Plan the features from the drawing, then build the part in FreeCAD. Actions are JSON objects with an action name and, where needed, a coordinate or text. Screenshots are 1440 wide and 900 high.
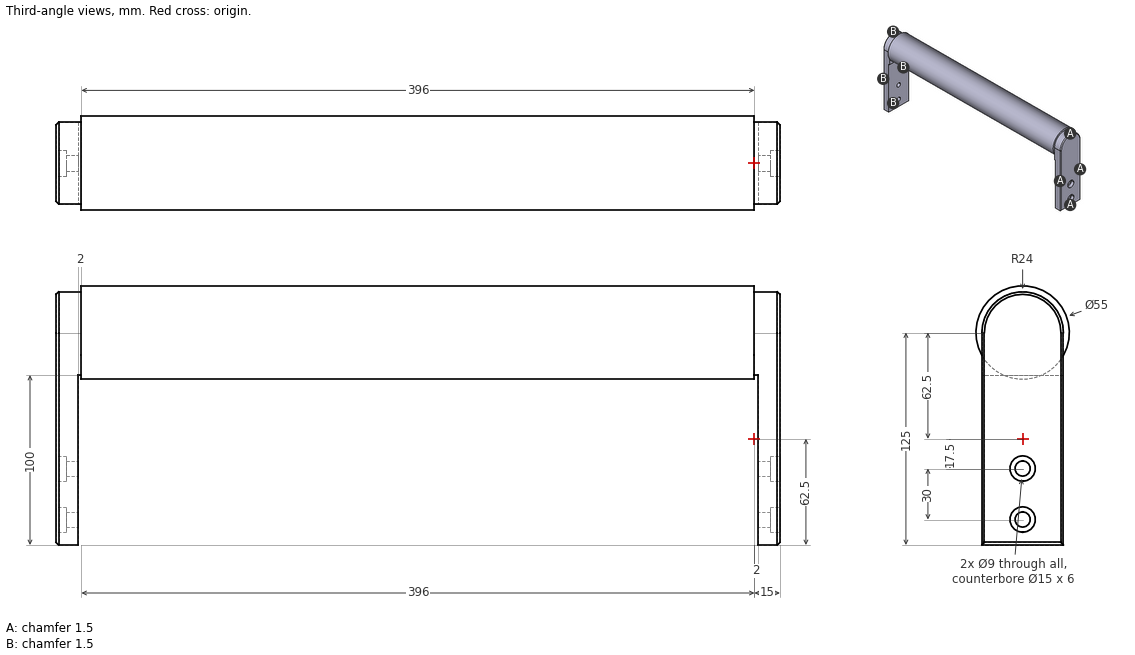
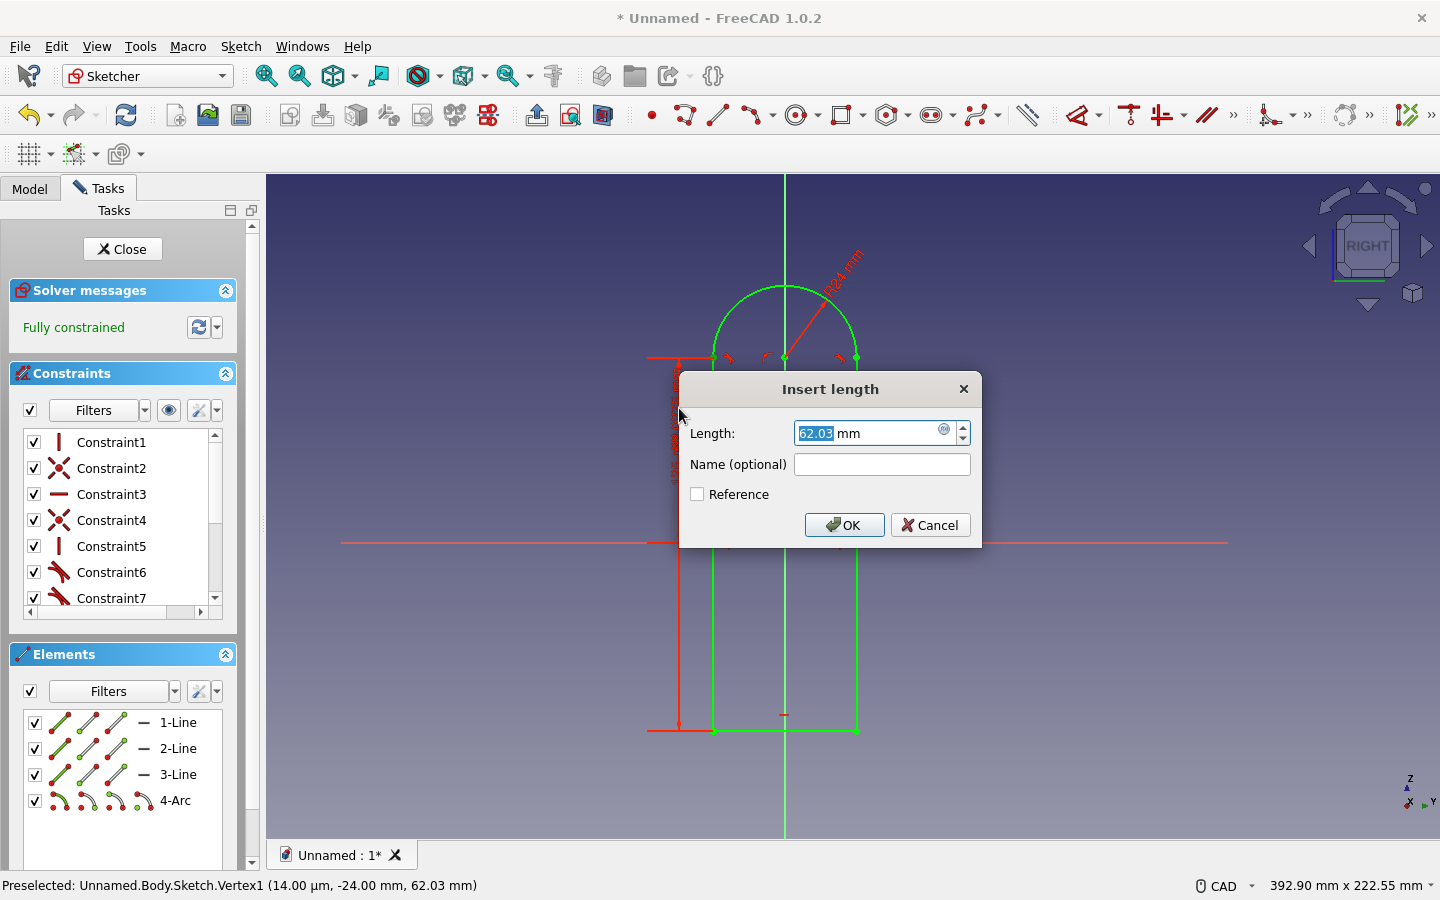
{"action": "type", "text": "62.5"}
{"action": "key", "text": "Return"}
{"action": "key", "text": "Escape"}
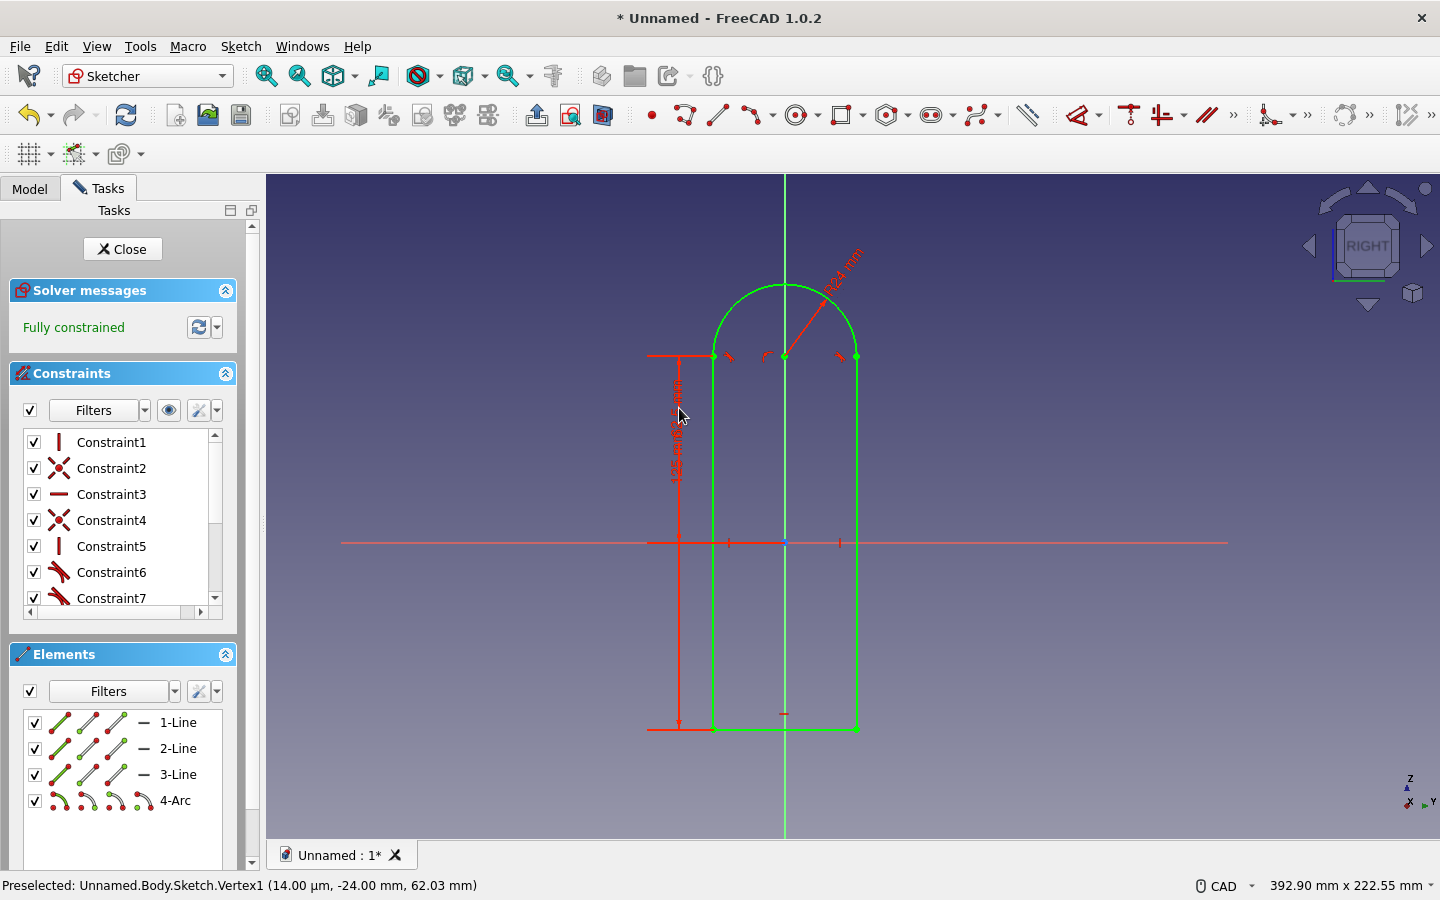
{"action": "left_click", "coordinate": [123, 249]}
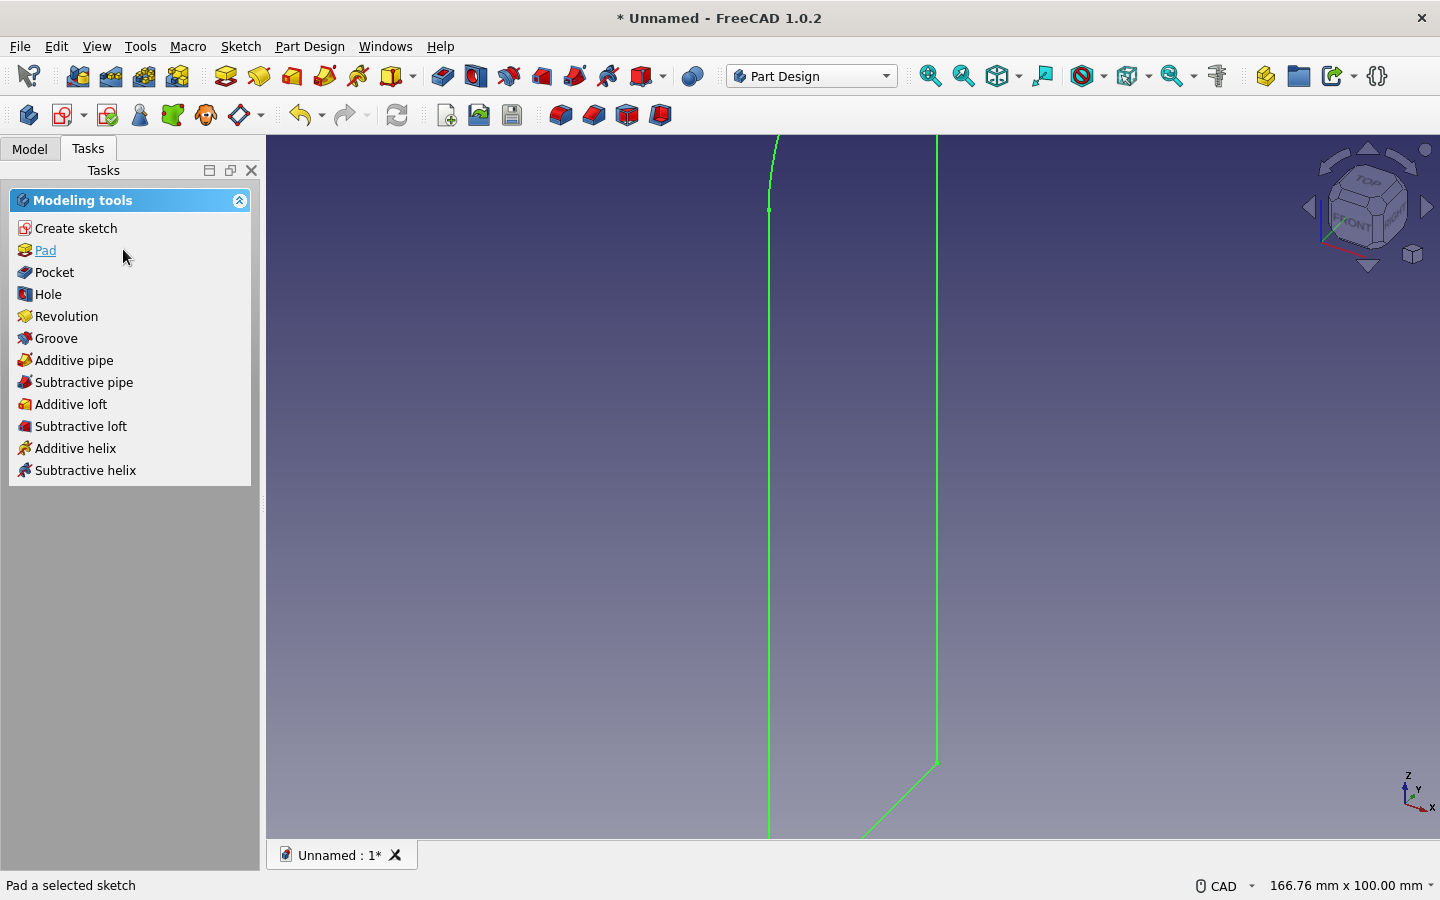
{"action": "left_click", "coordinate": [226, 76]}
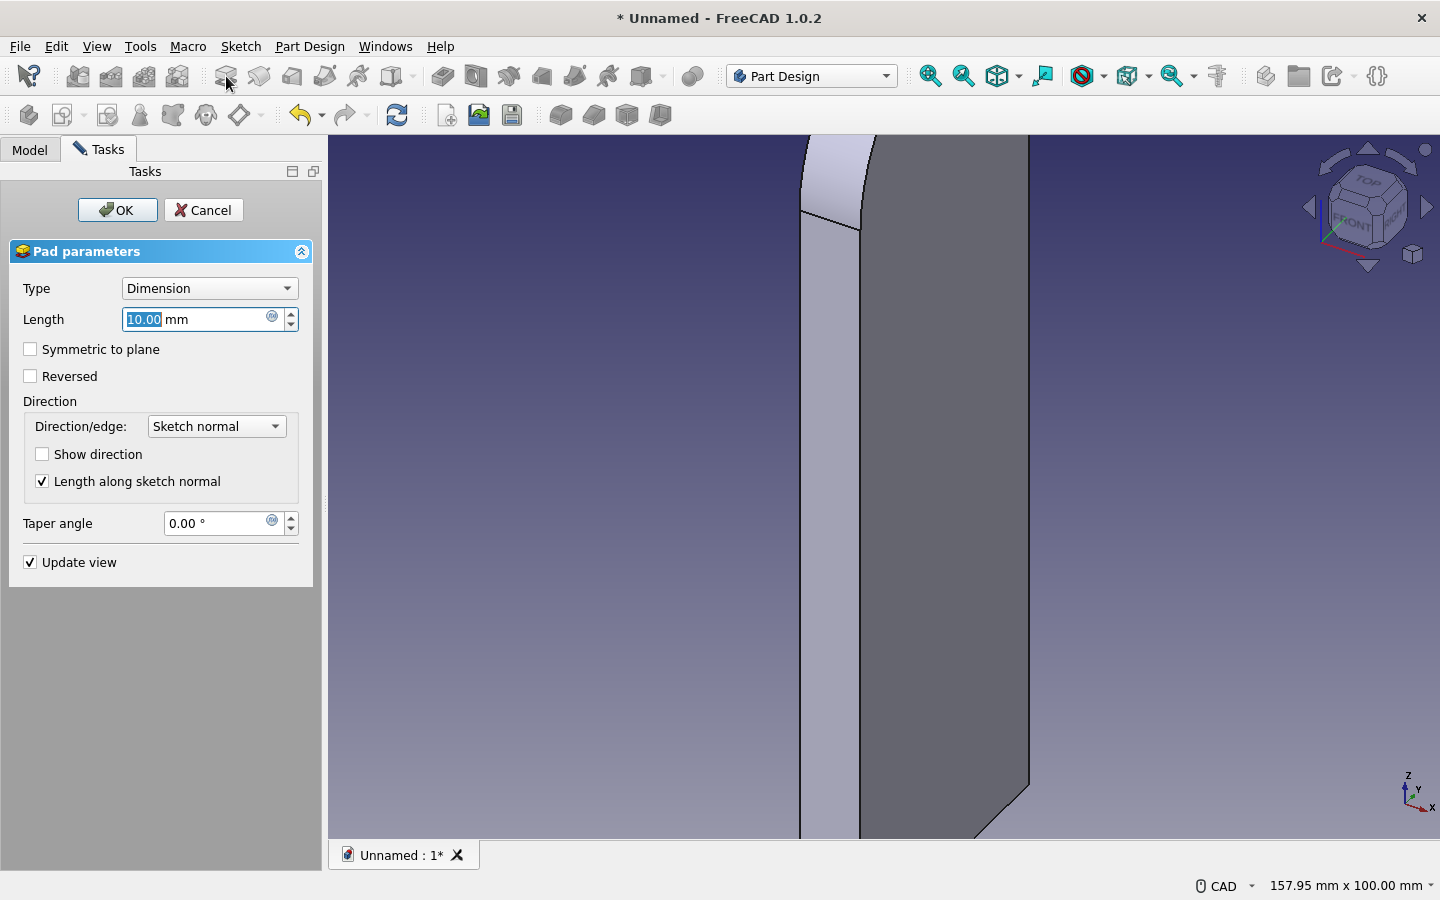
{"action": "type", "text": "15"}
{"action": "key", "text": "Tab"}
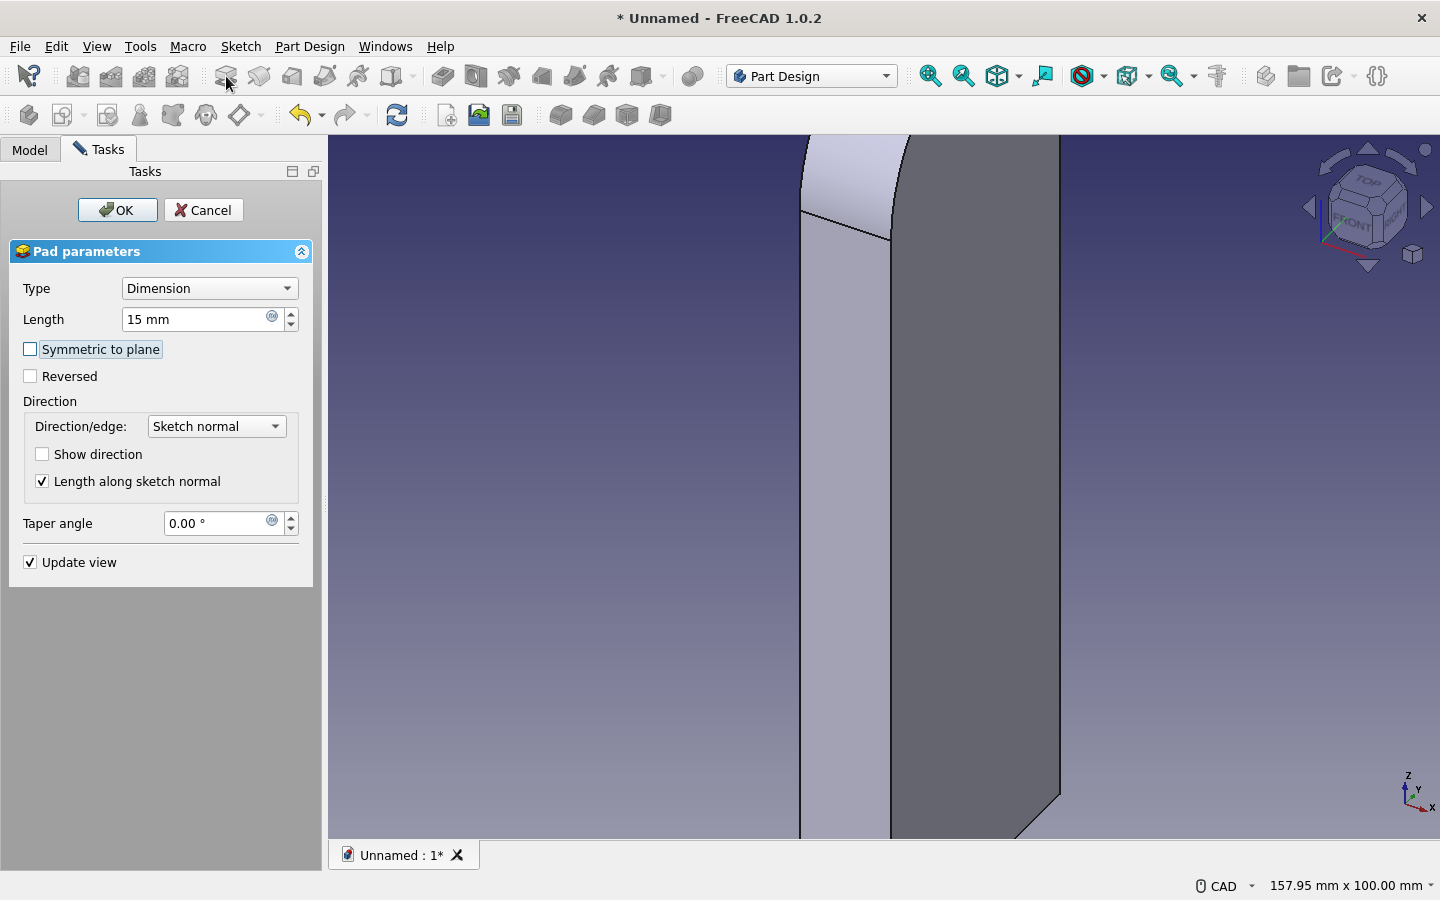
{"action": "left_click", "coordinate": [118, 210]}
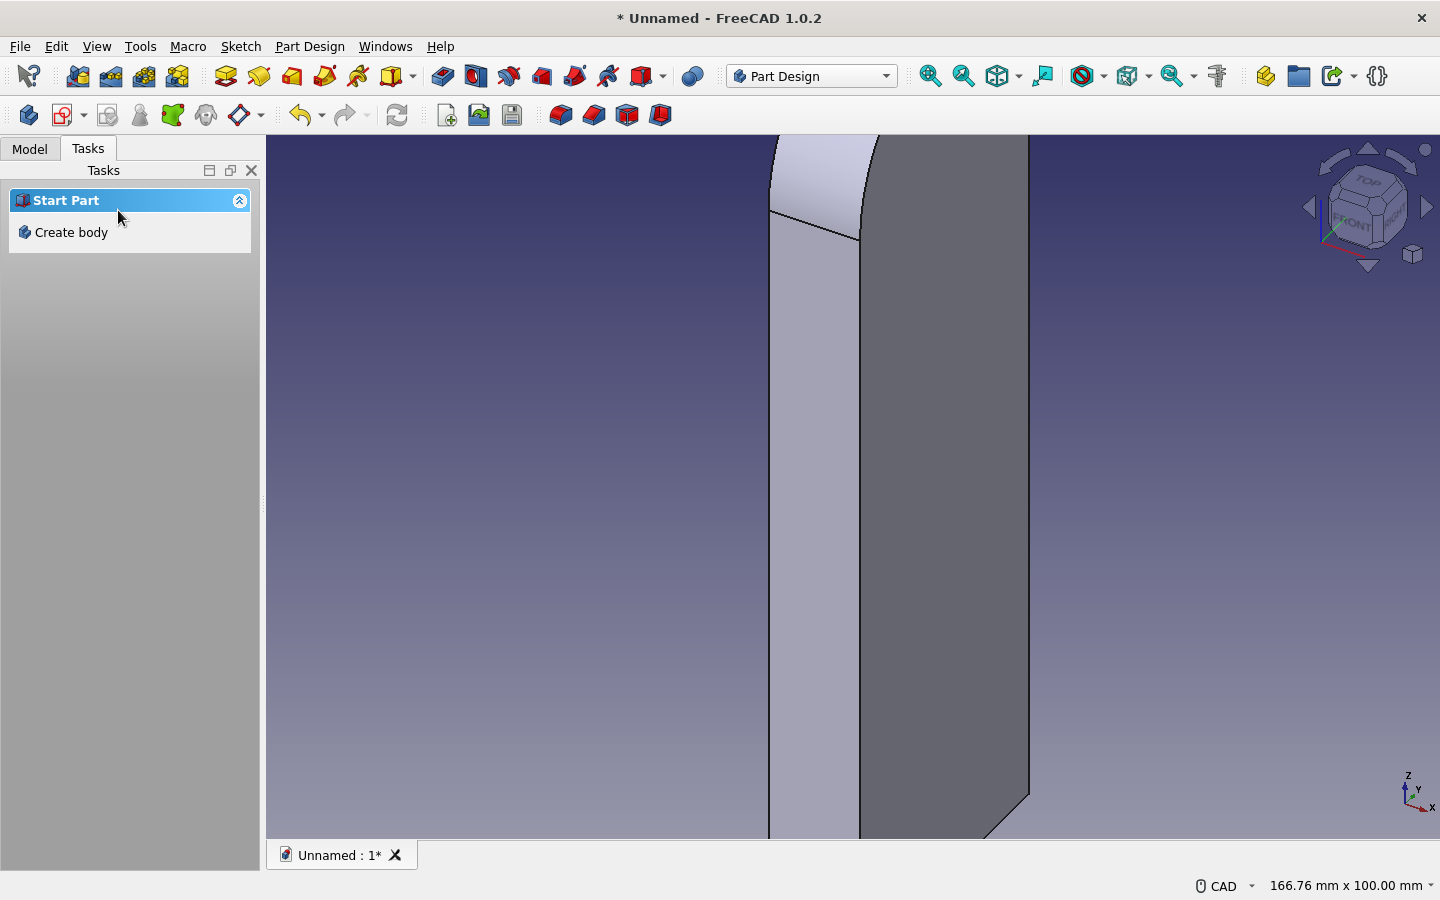
{"action": "left_click", "coordinate": [931, 76]}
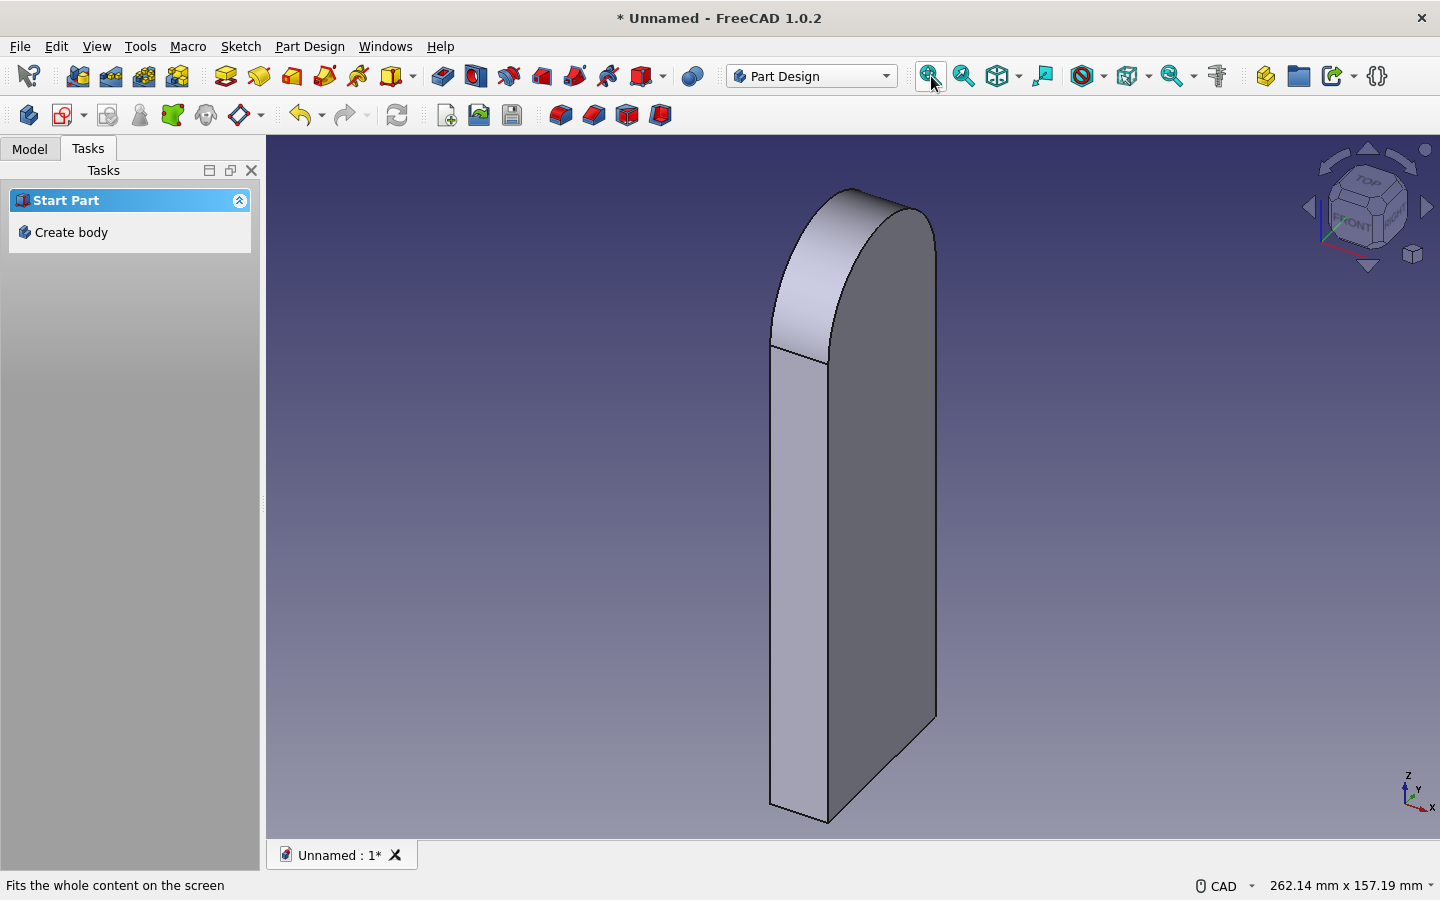
{"action": "key", "text": "6"}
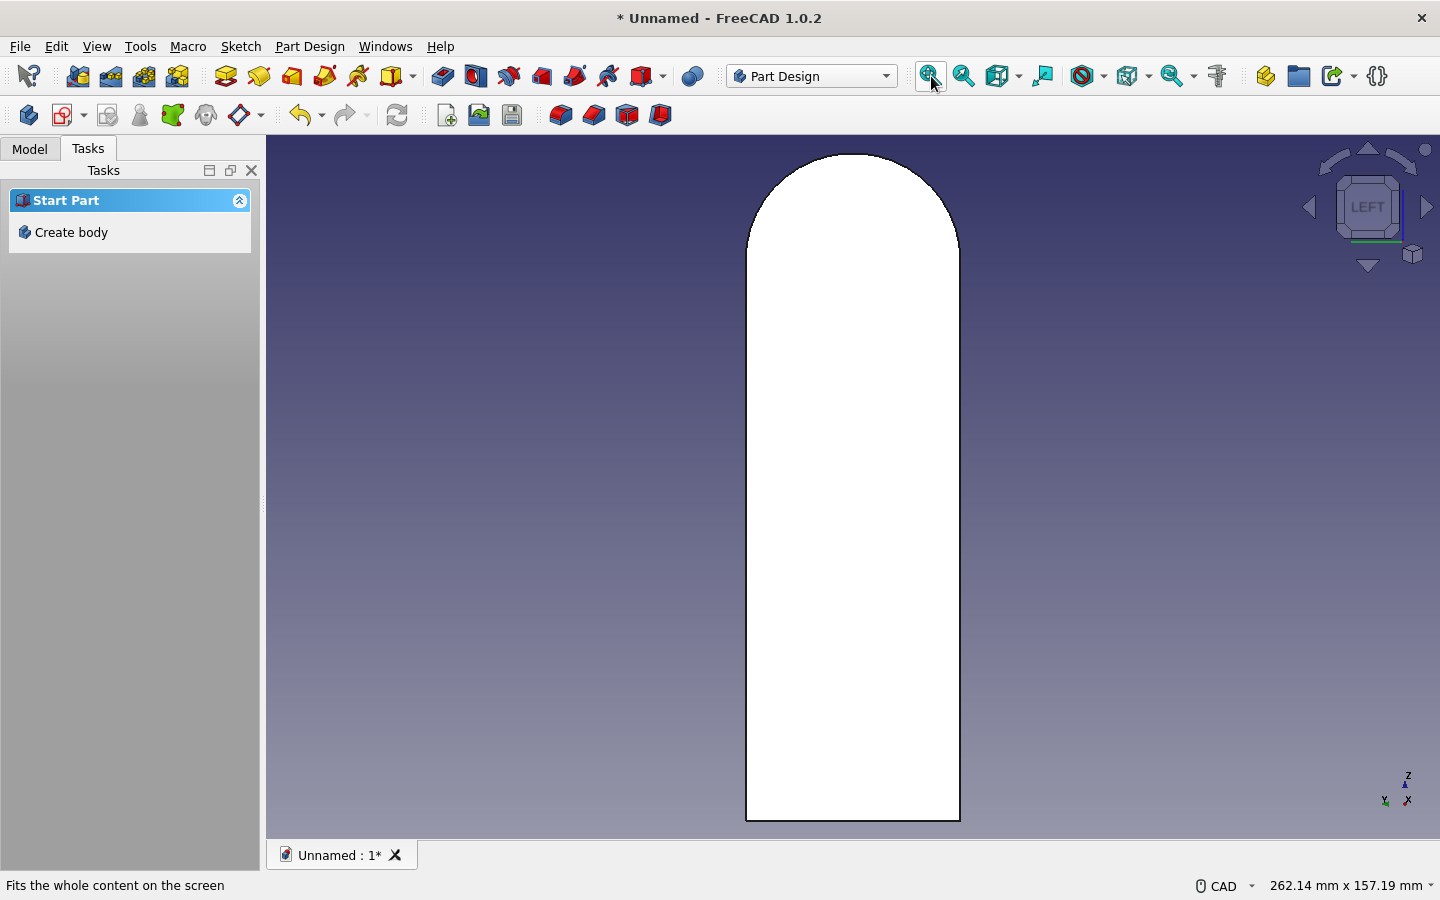
{"action": "left_click", "coordinate": [853, 677]}